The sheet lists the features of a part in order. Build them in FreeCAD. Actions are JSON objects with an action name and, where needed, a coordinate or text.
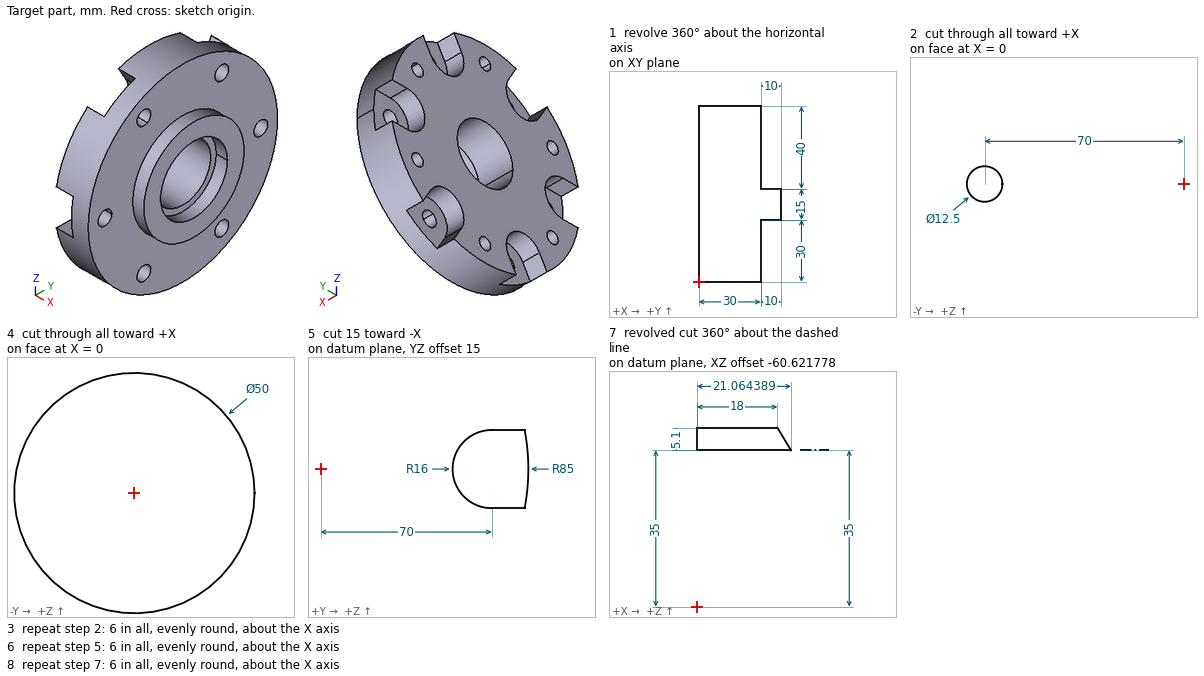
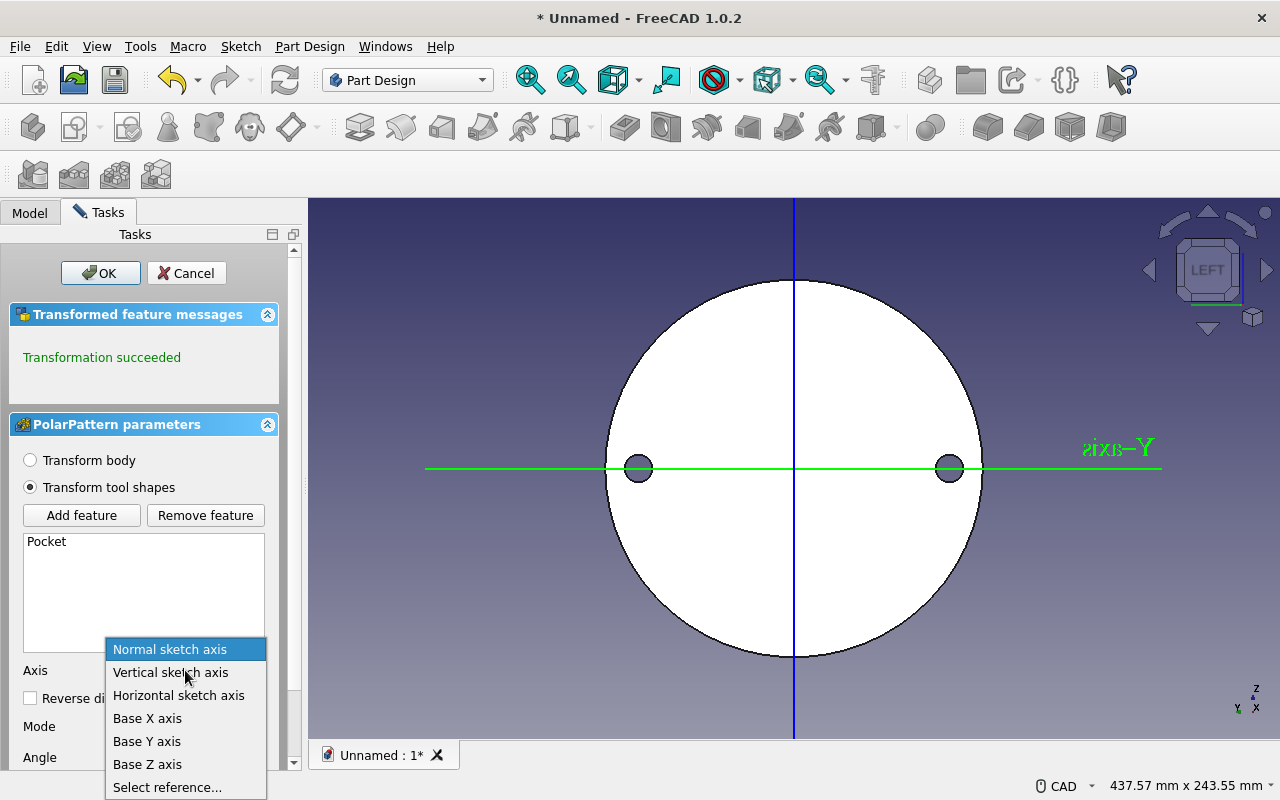
{"action": "left_click", "coordinate": [184, 718]}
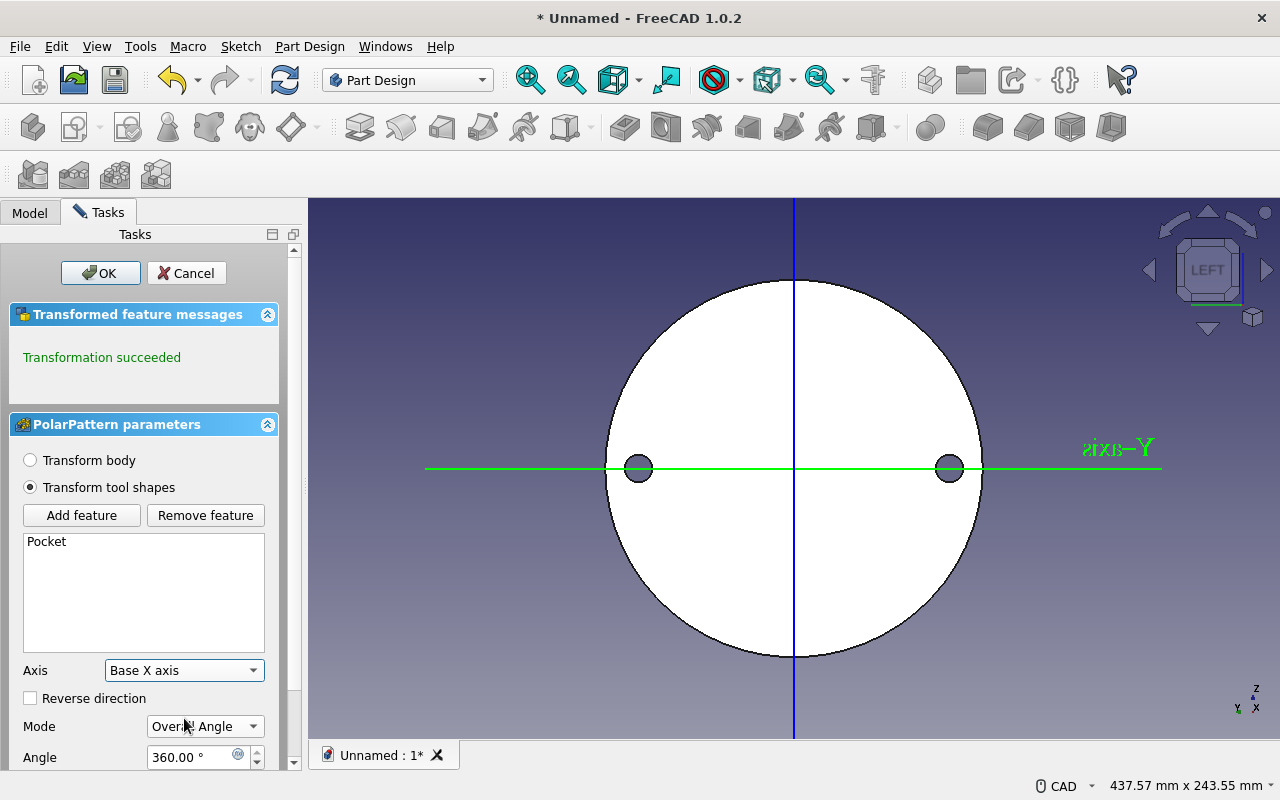
{"action": "scroll", "coordinate": [294, 507], "scroll_direction": "down", "scroll_amount": 2}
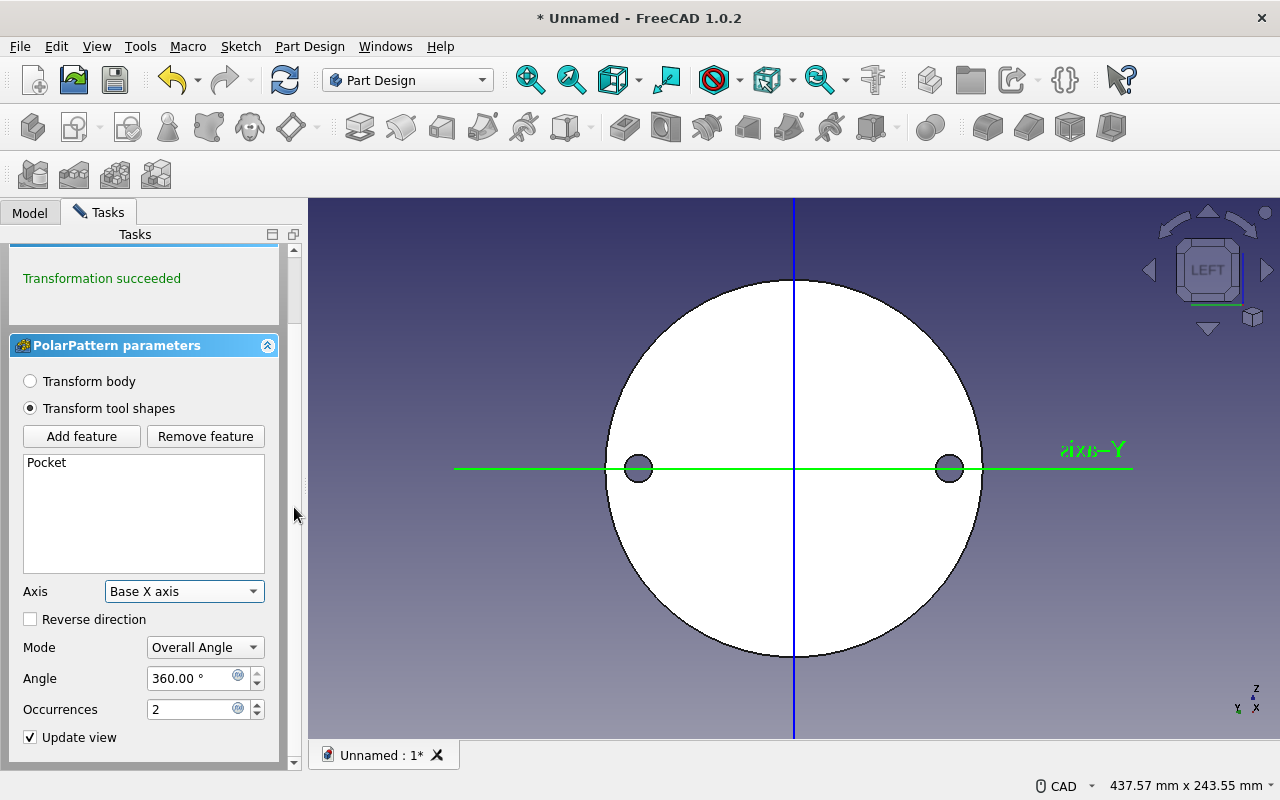
{"action": "triple_click", "coordinate": [199, 710]}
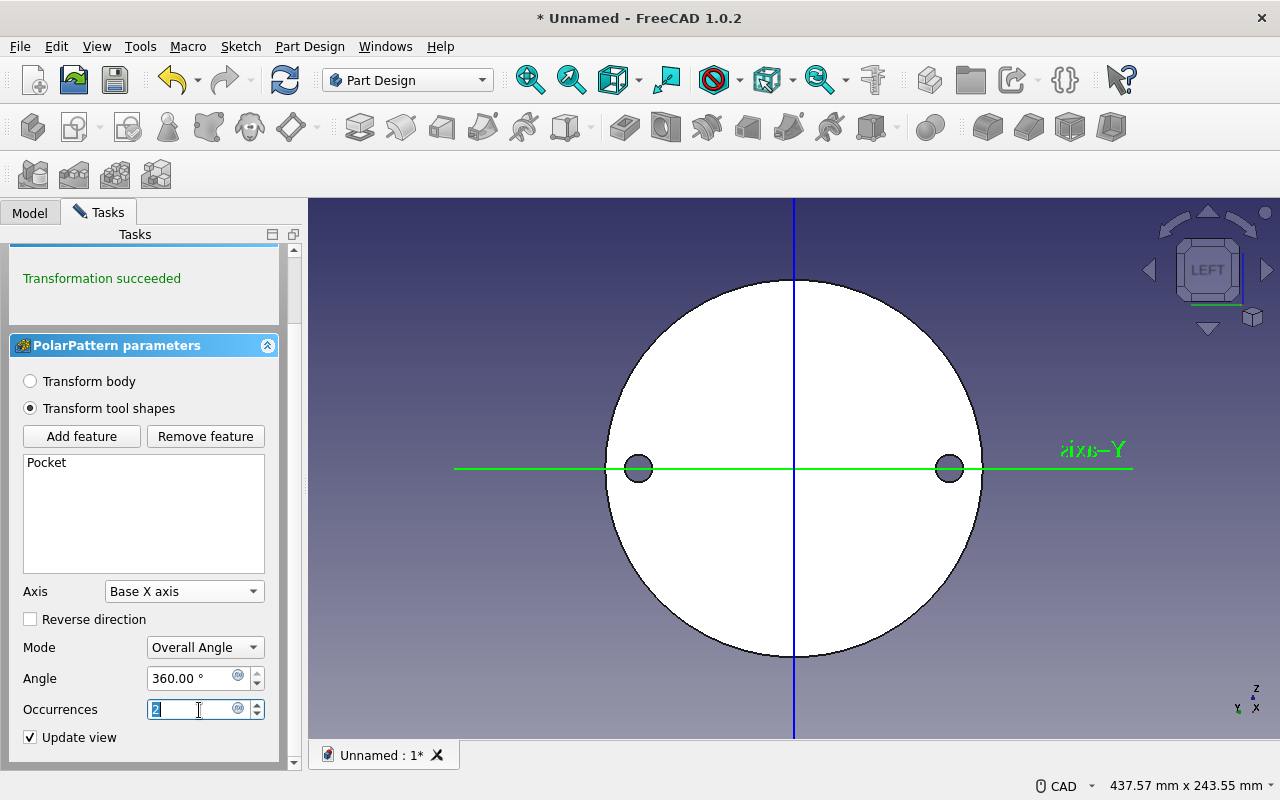
{"action": "type", "text": "6"}
{"action": "key", "text": "Tab"}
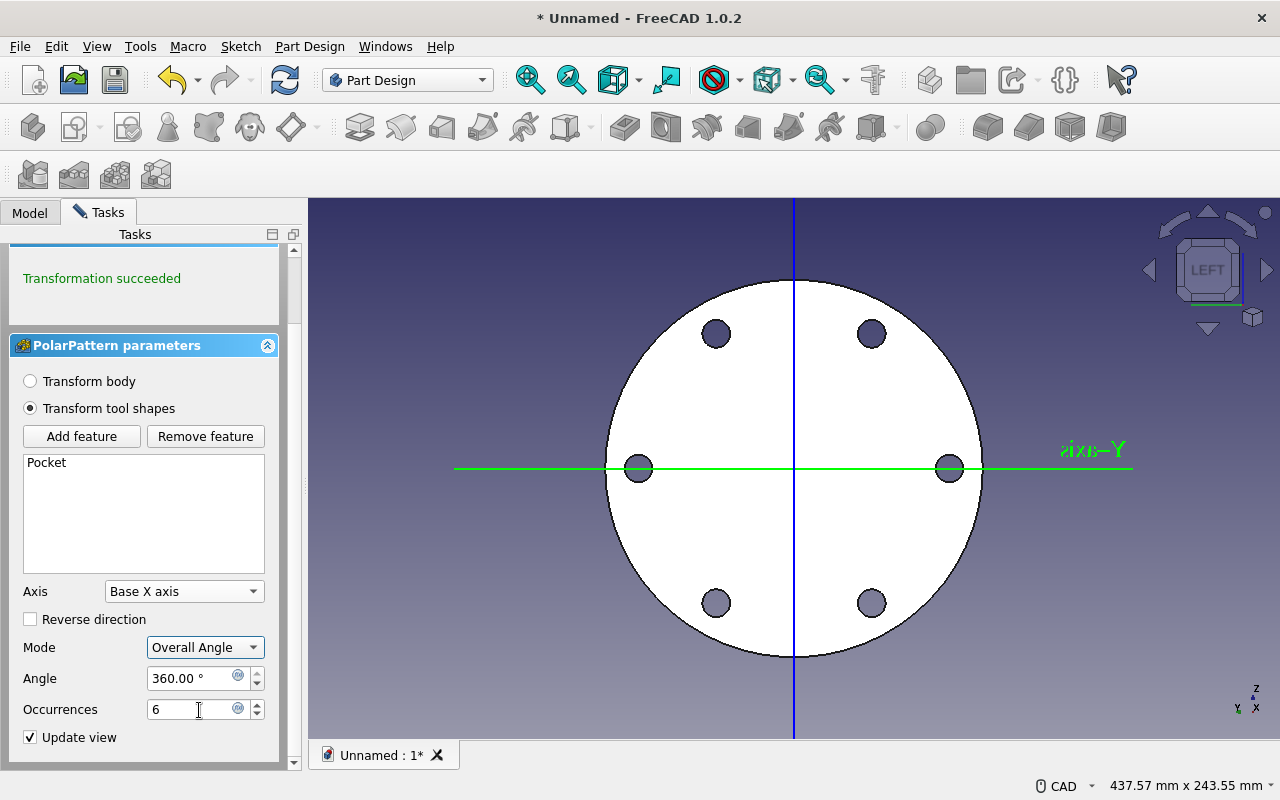
{"action": "scroll", "coordinate": [294, 507], "scroll_direction": "up", "scroll_amount": 3}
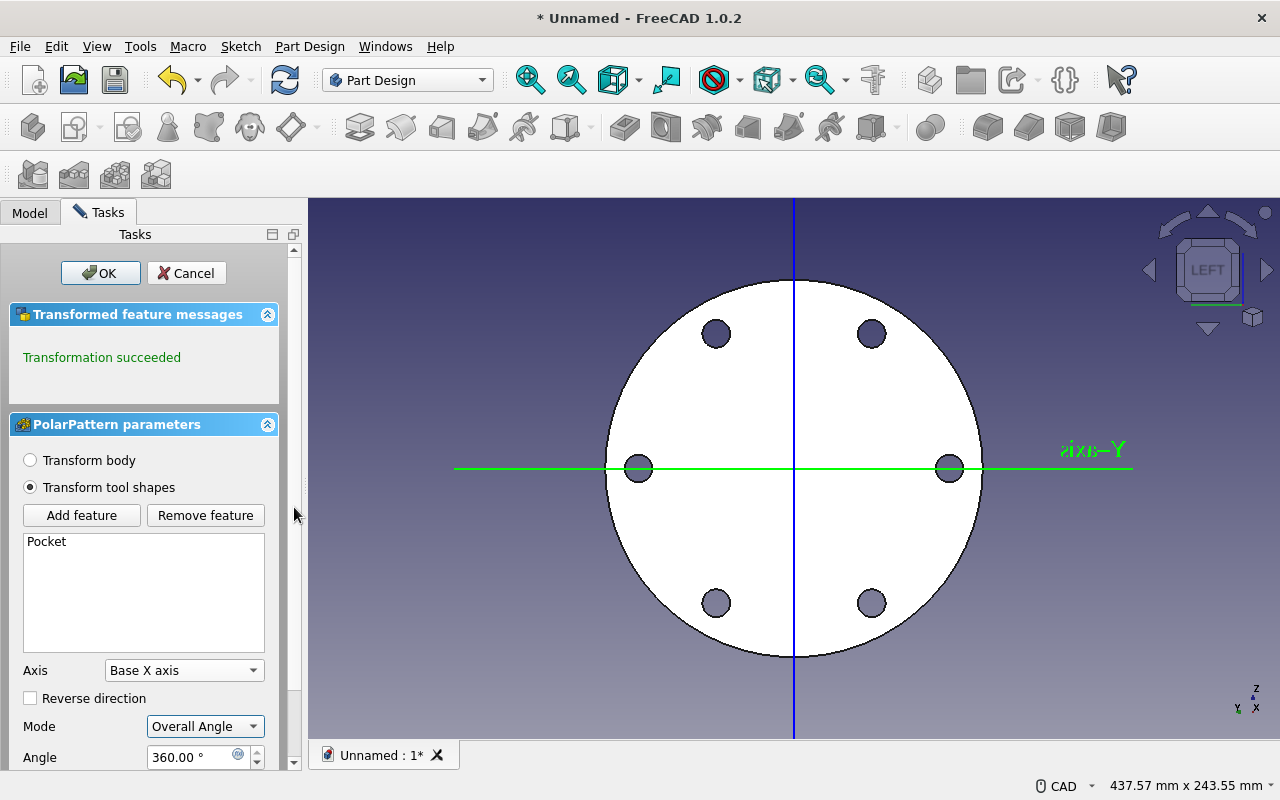
{"action": "left_click", "coordinate": [101, 273]}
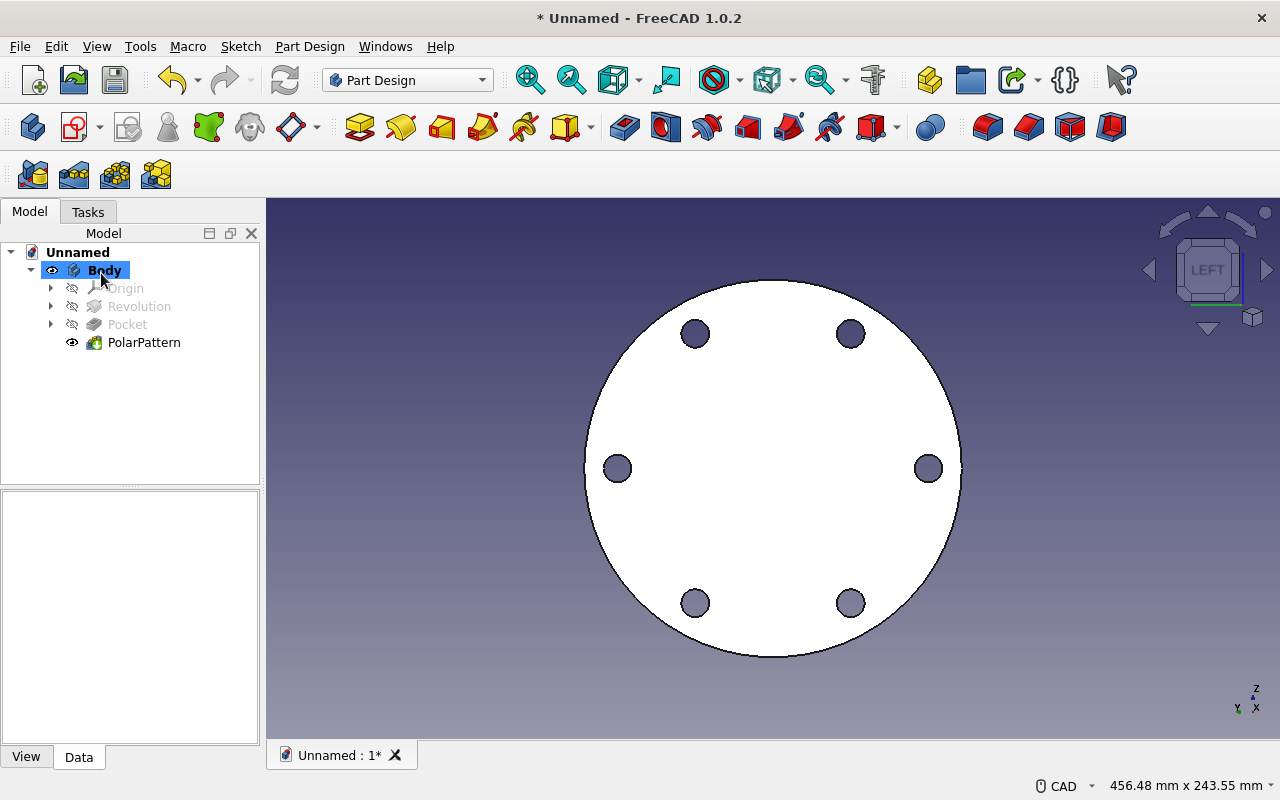
{"action": "left_click", "coordinate": [773, 467]}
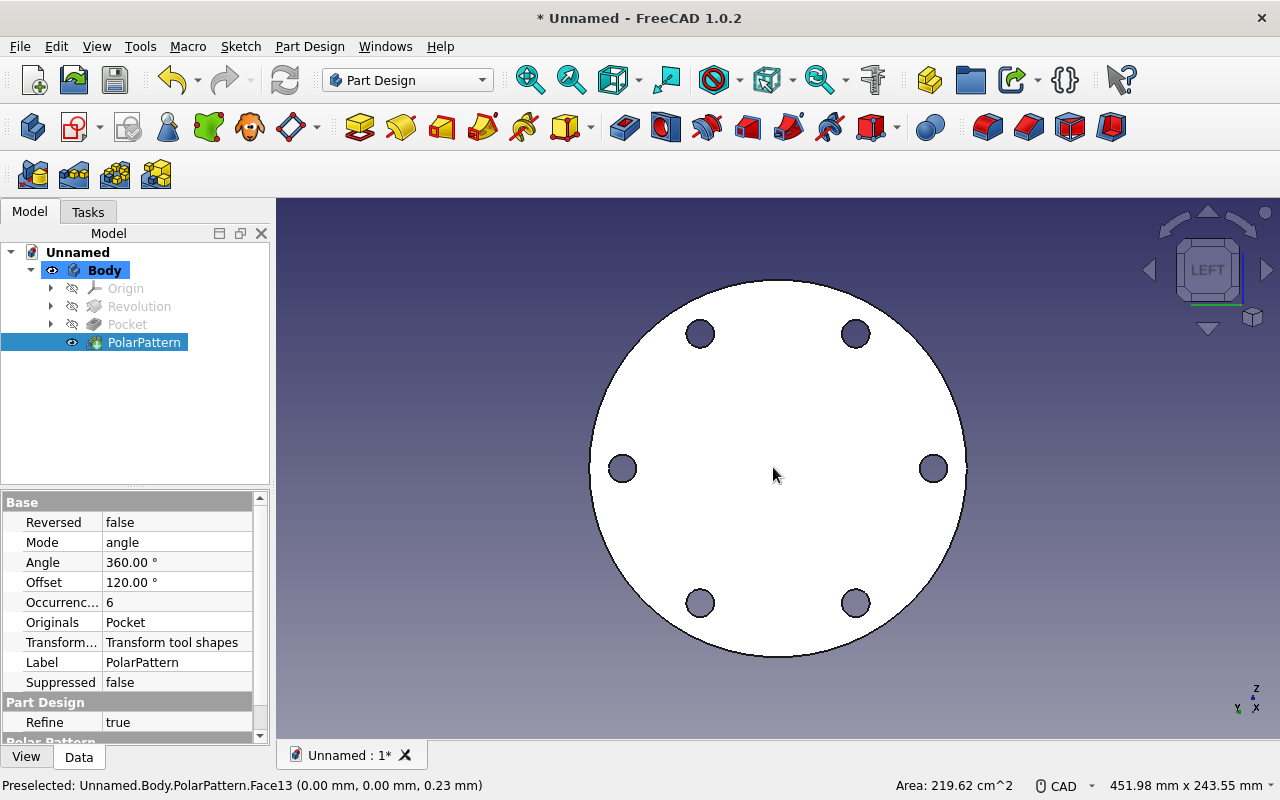
{"action": "left_click", "coordinate": [74, 128]}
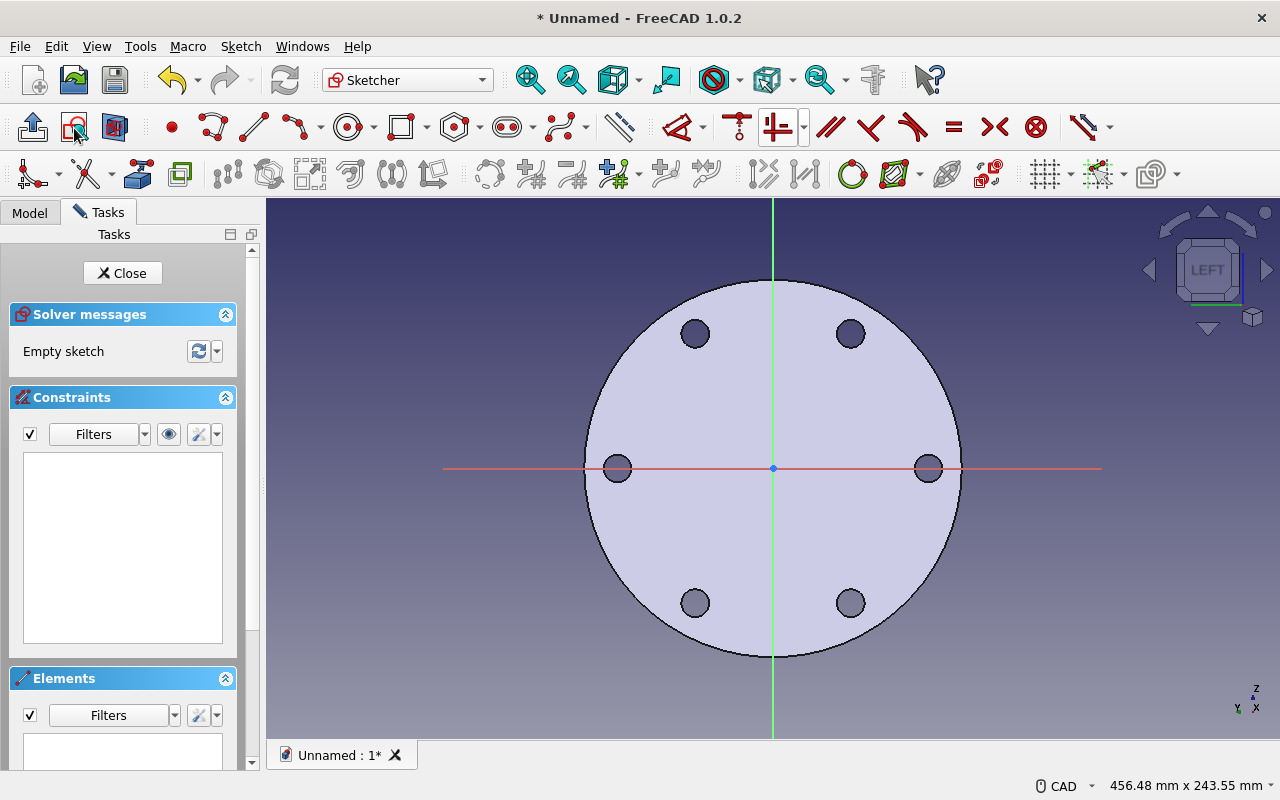
{"action": "scroll", "coordinate": [803, 469], "scroll_direction": "up", "scroll_amount": 6}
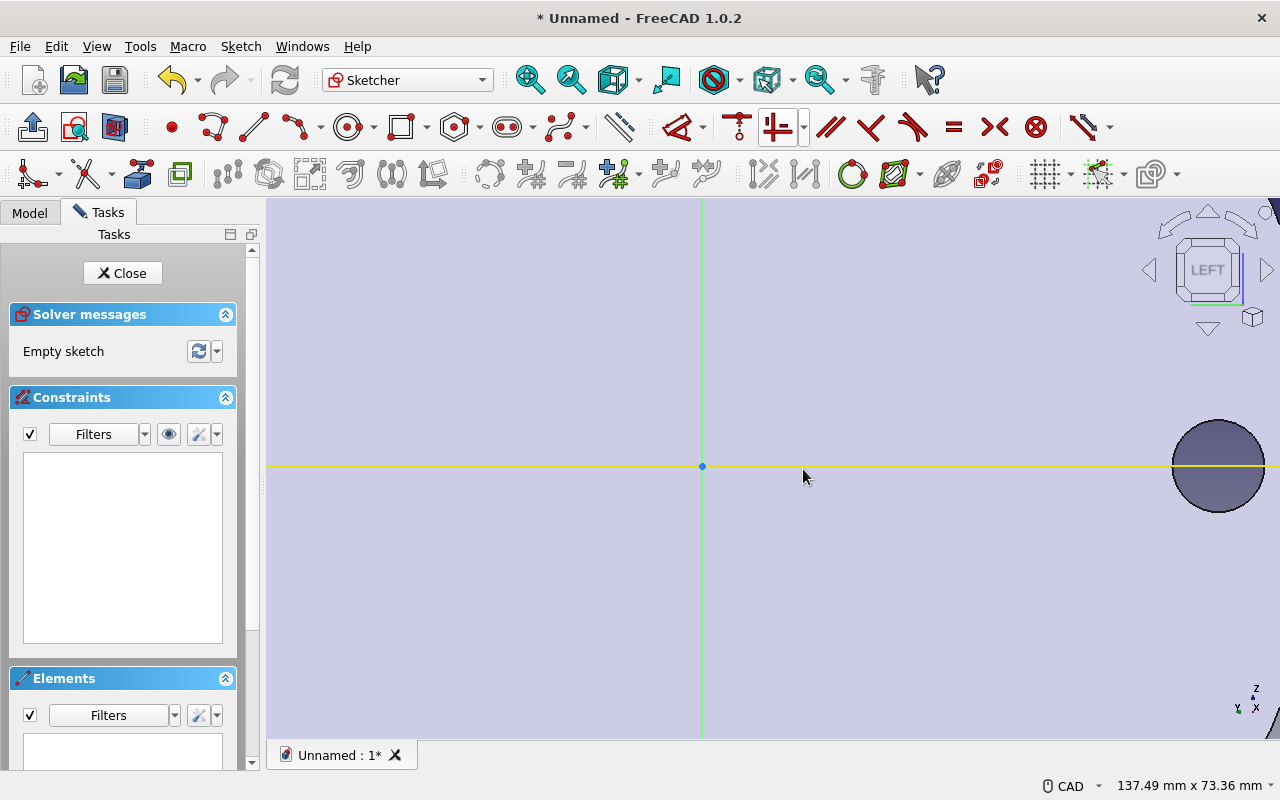
{"action": "left_click", "coordinate": [348, 128]}